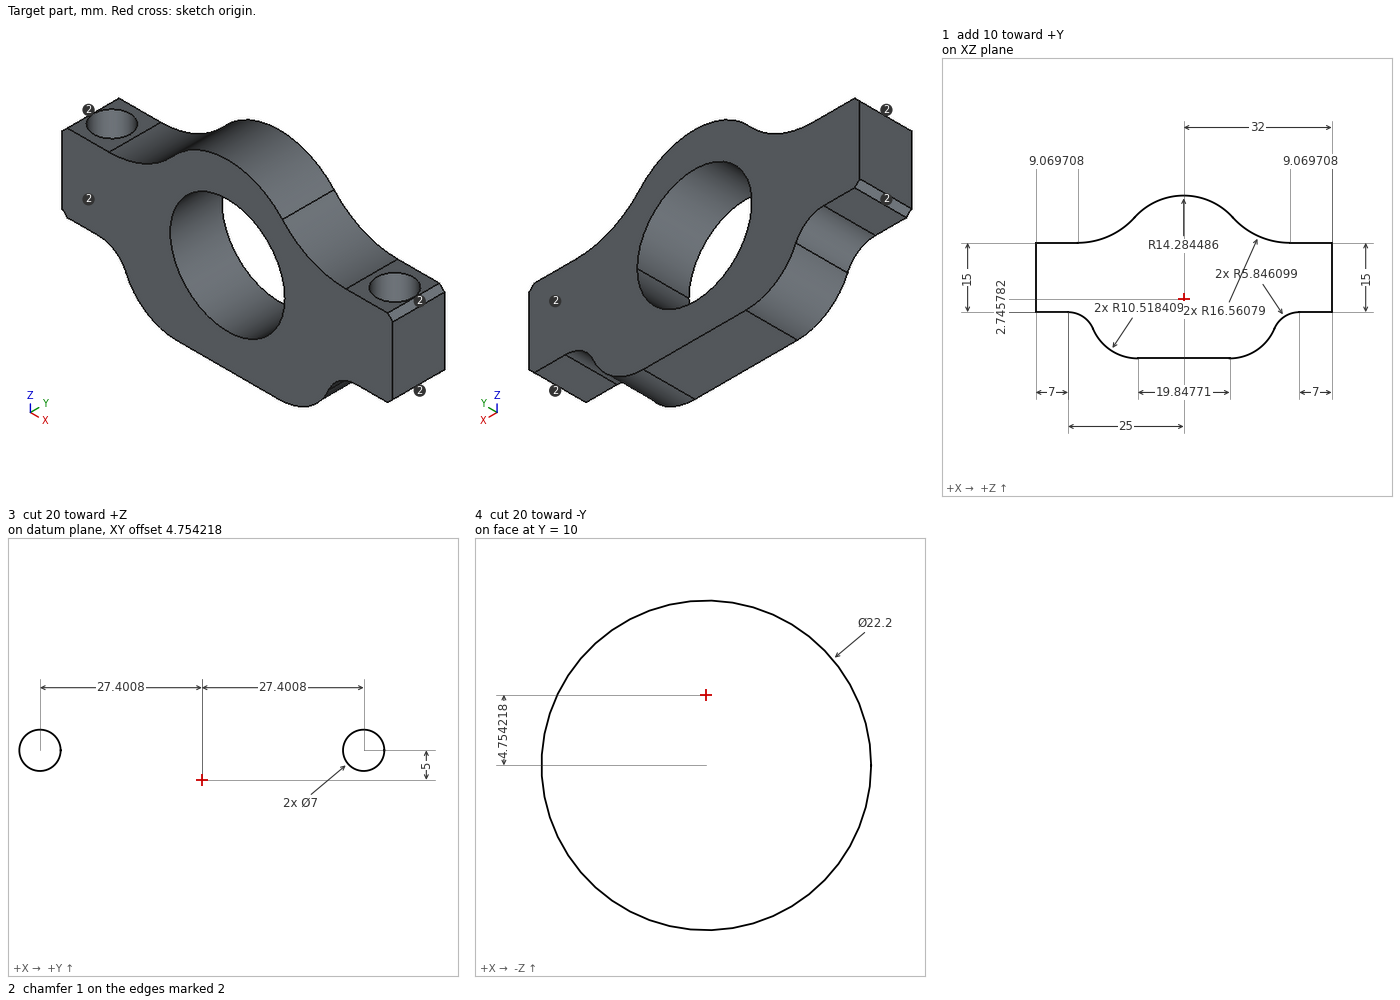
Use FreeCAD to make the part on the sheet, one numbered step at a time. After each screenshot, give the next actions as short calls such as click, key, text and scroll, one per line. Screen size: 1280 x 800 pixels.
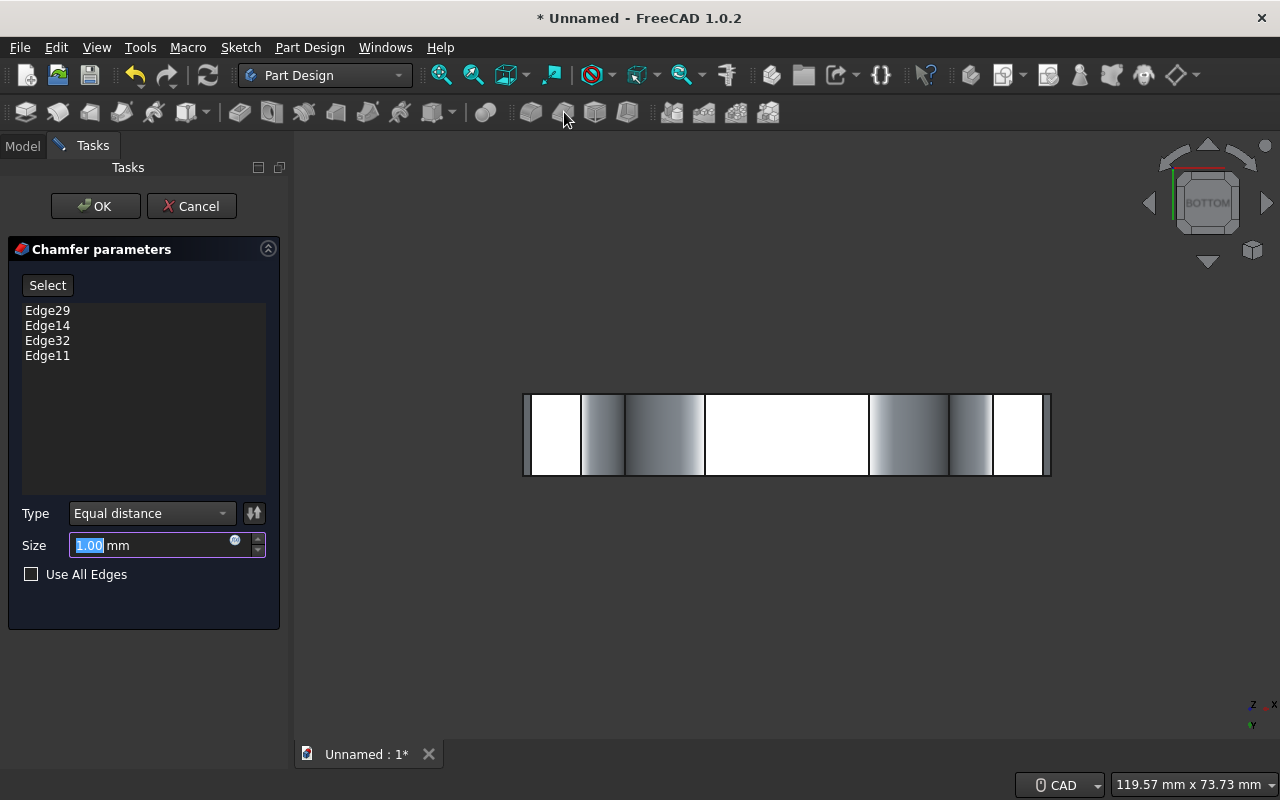
text(1)
key(Tab)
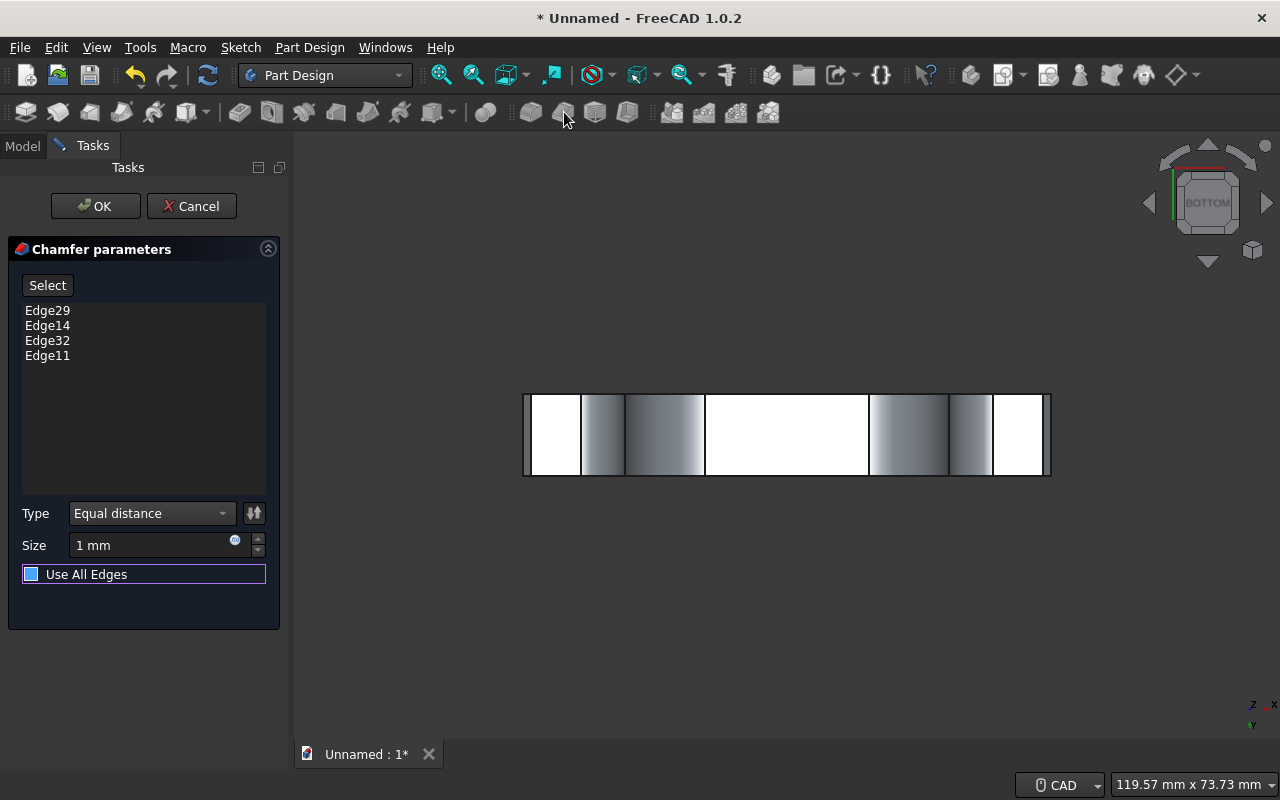
click(96, 206)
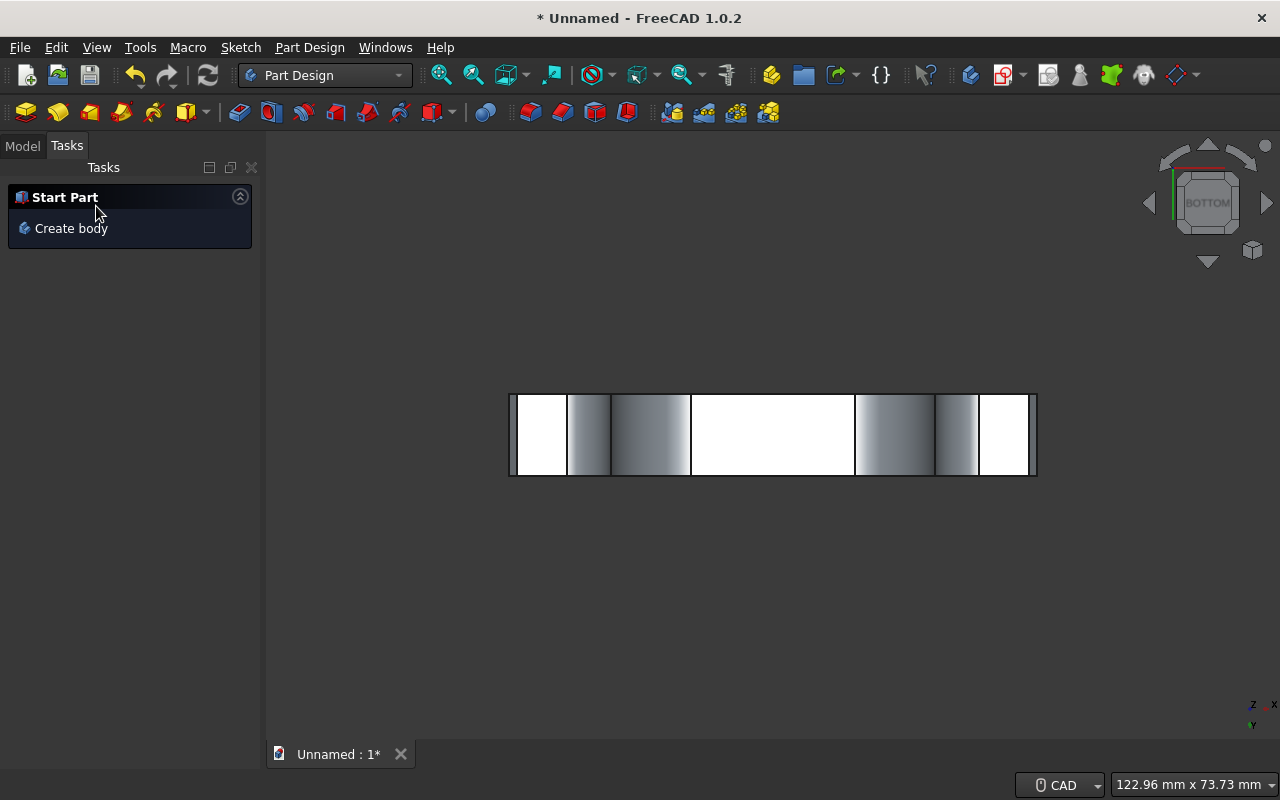
click(23, 145)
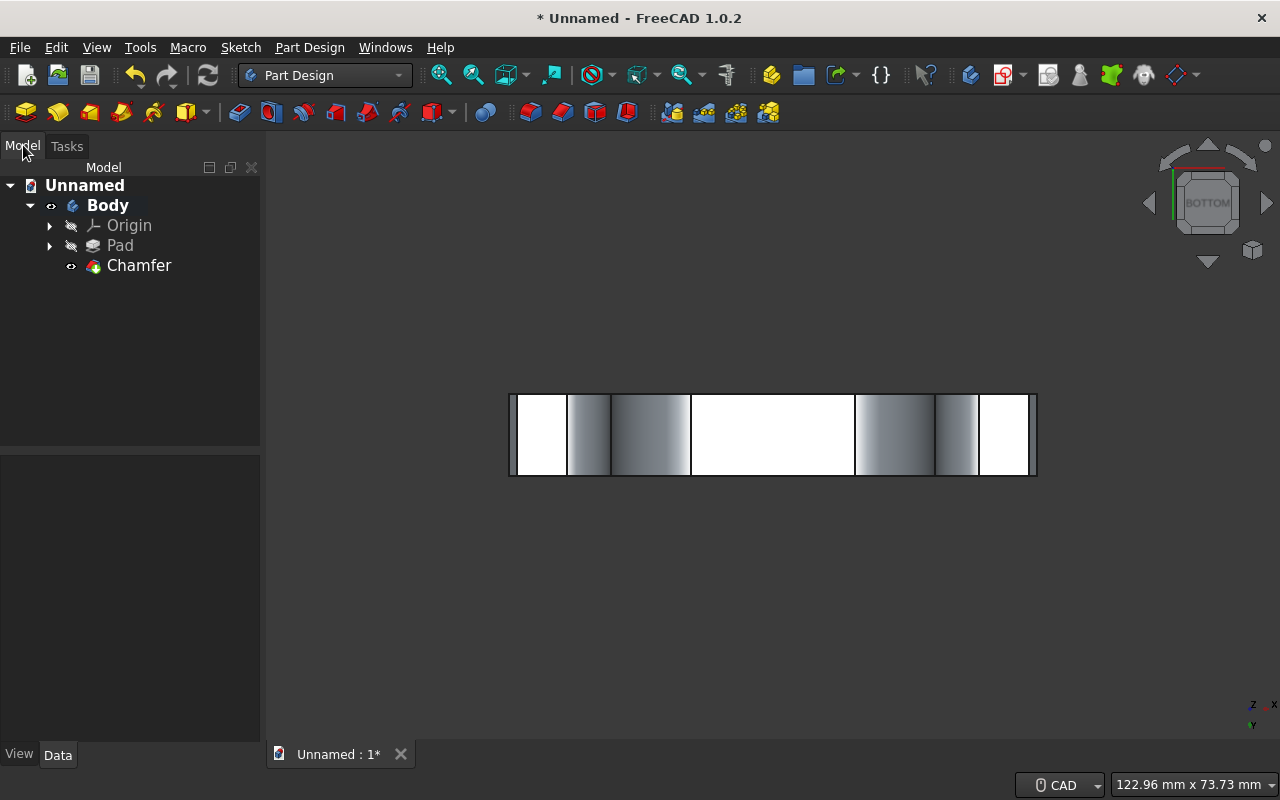
click(50, 226)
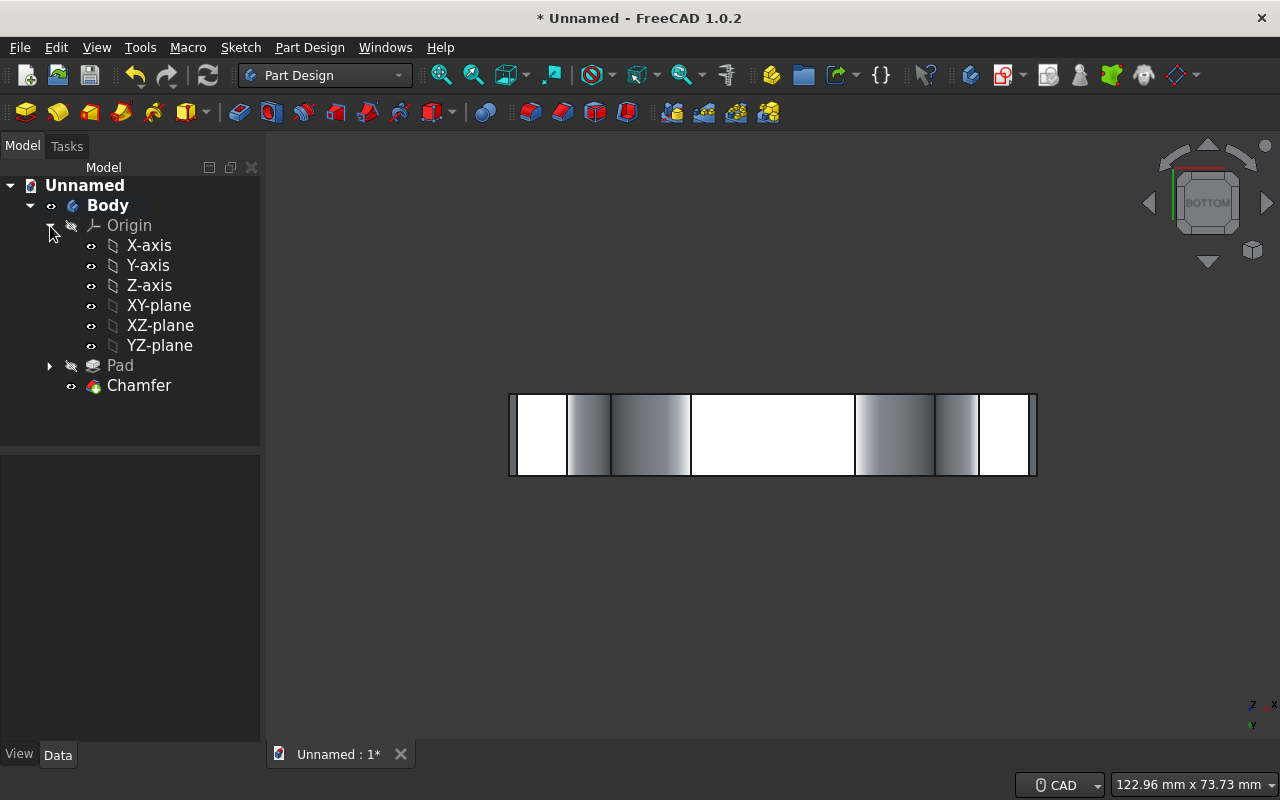
click(136, 306)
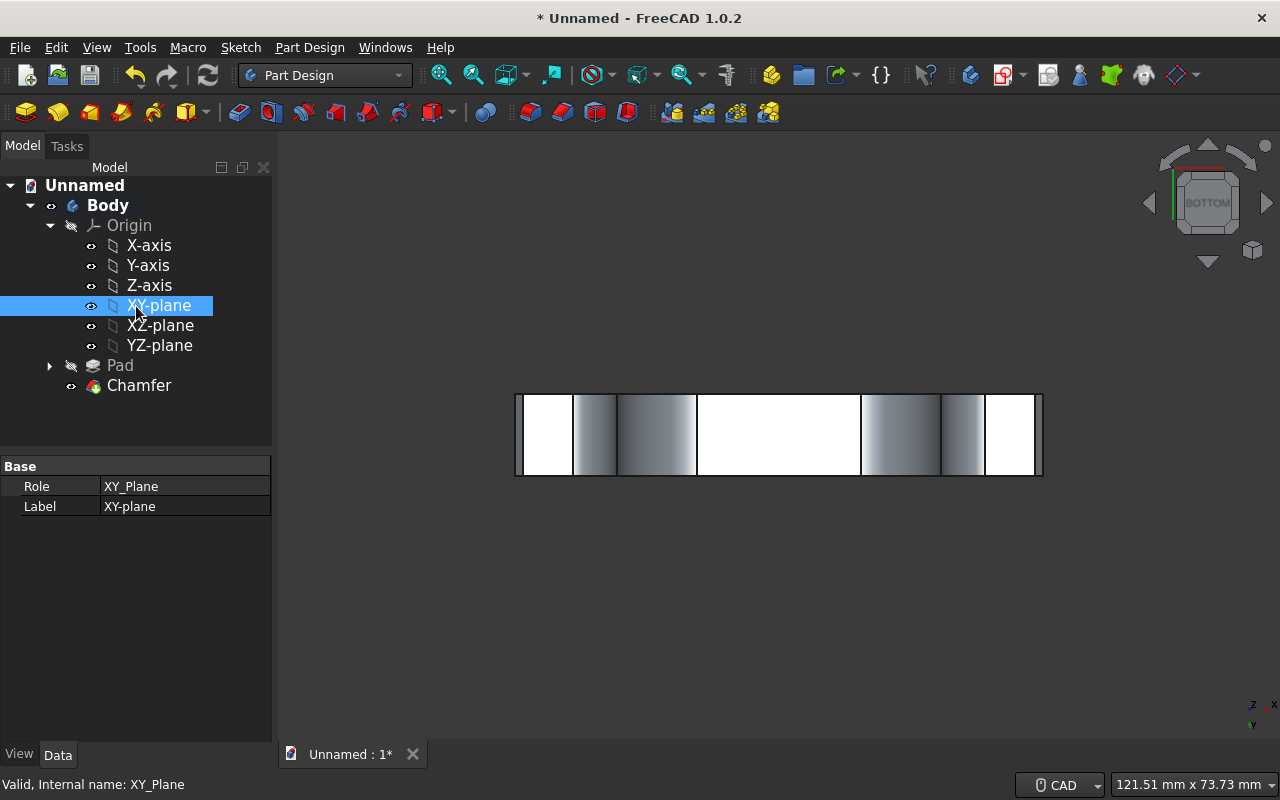
click(1176, 76)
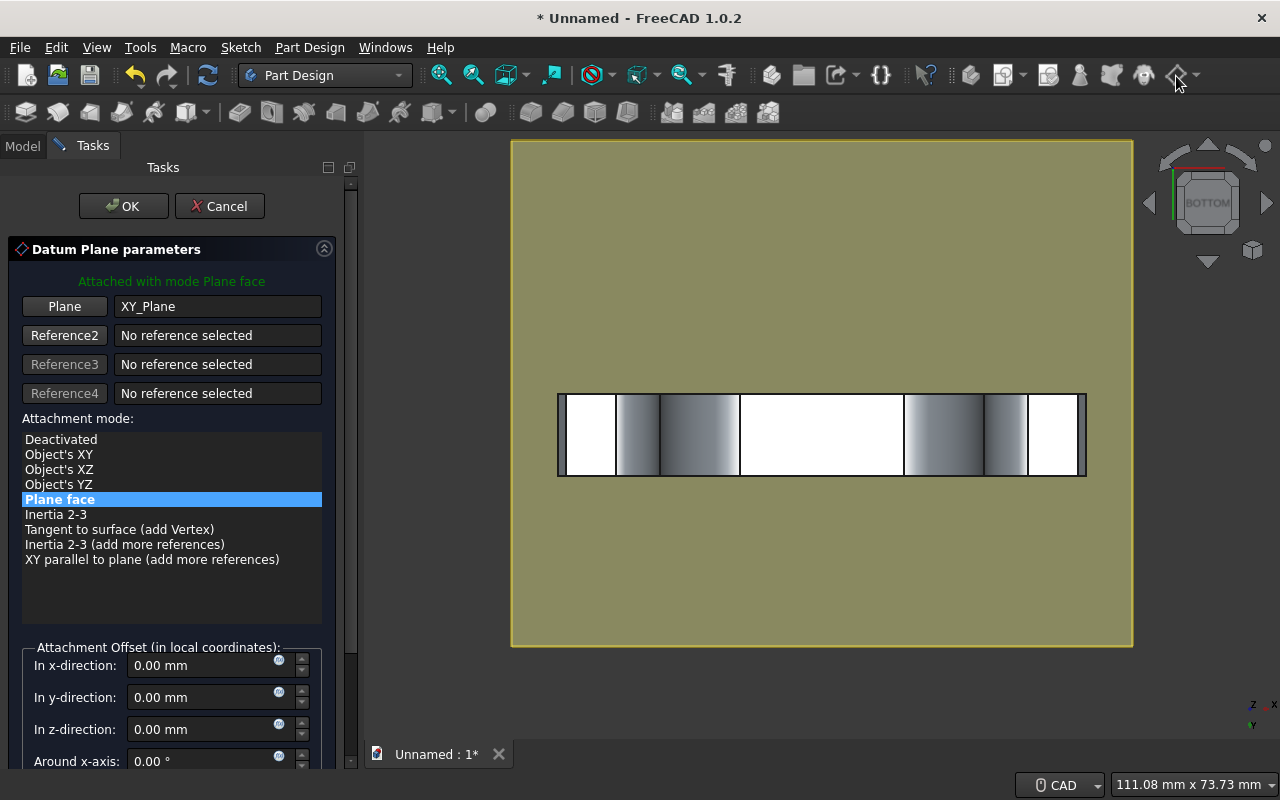
triple_click(210, 729)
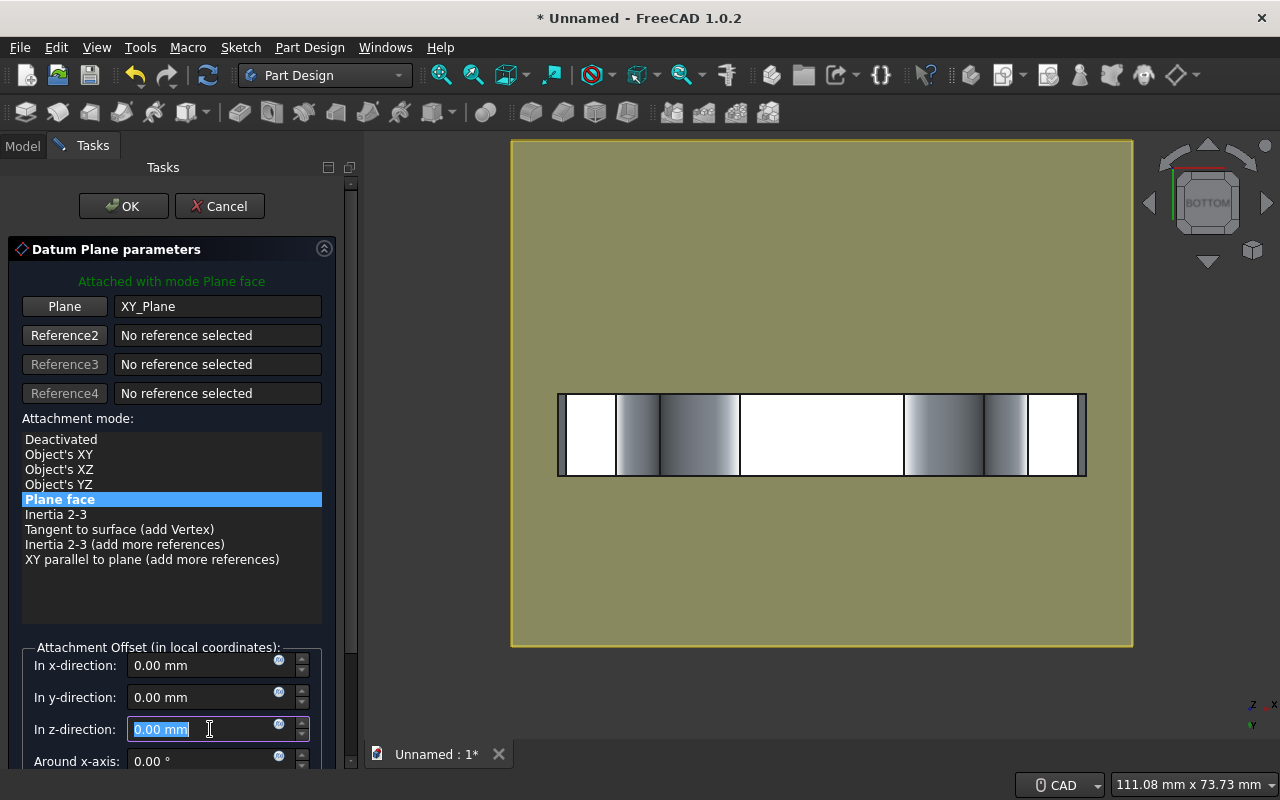
text(4.754218)
key(Tab)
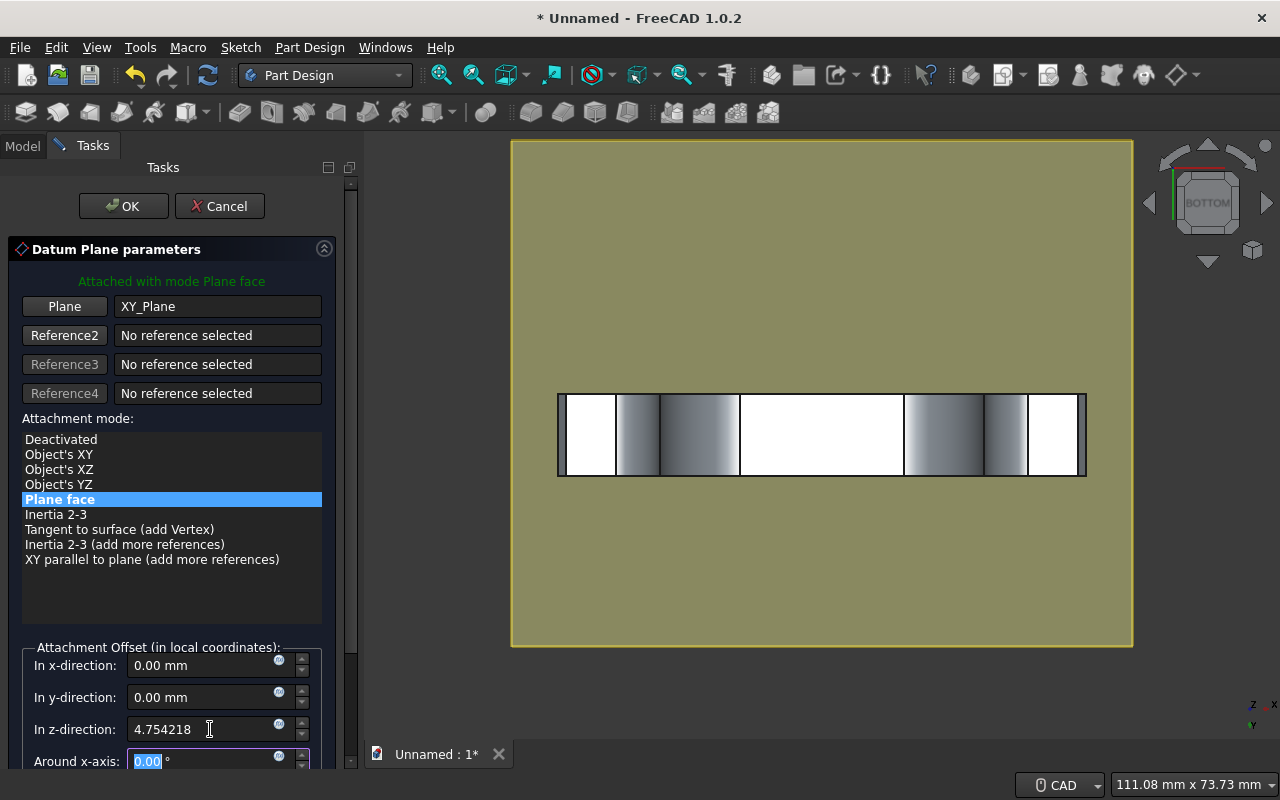
click(124, 206)